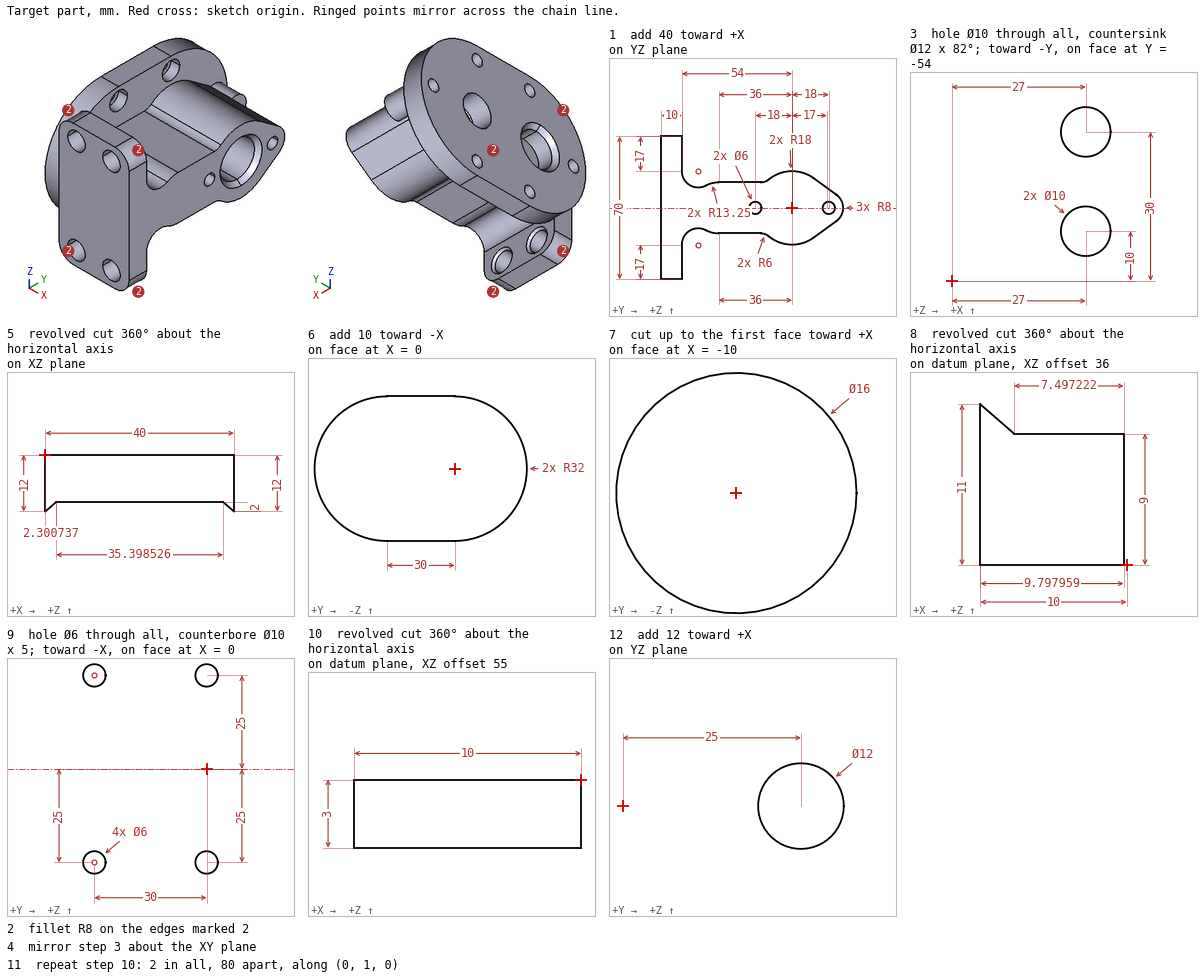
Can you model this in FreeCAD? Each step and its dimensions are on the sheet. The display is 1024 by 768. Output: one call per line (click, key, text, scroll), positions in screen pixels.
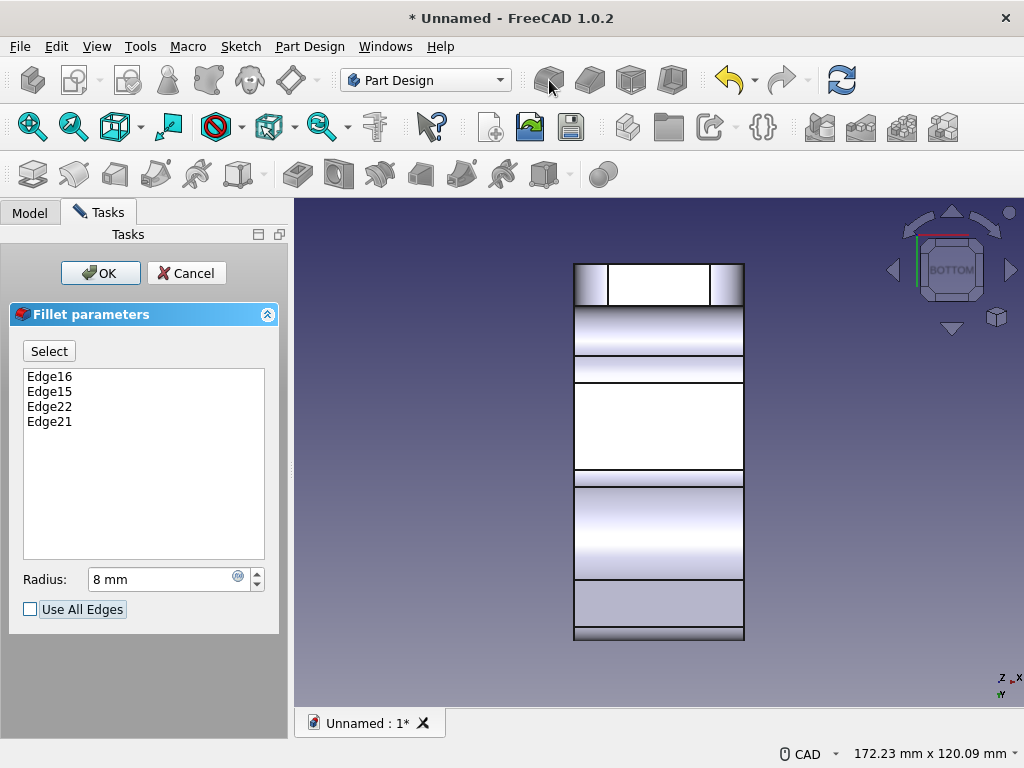
click(101, 273)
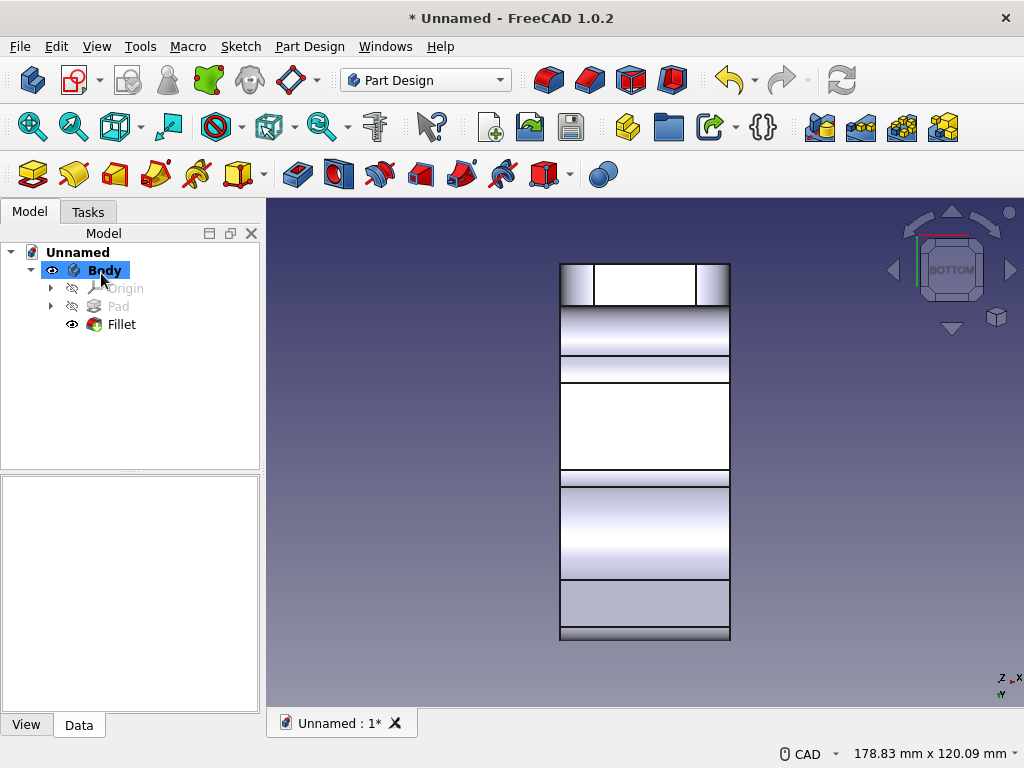
key(4)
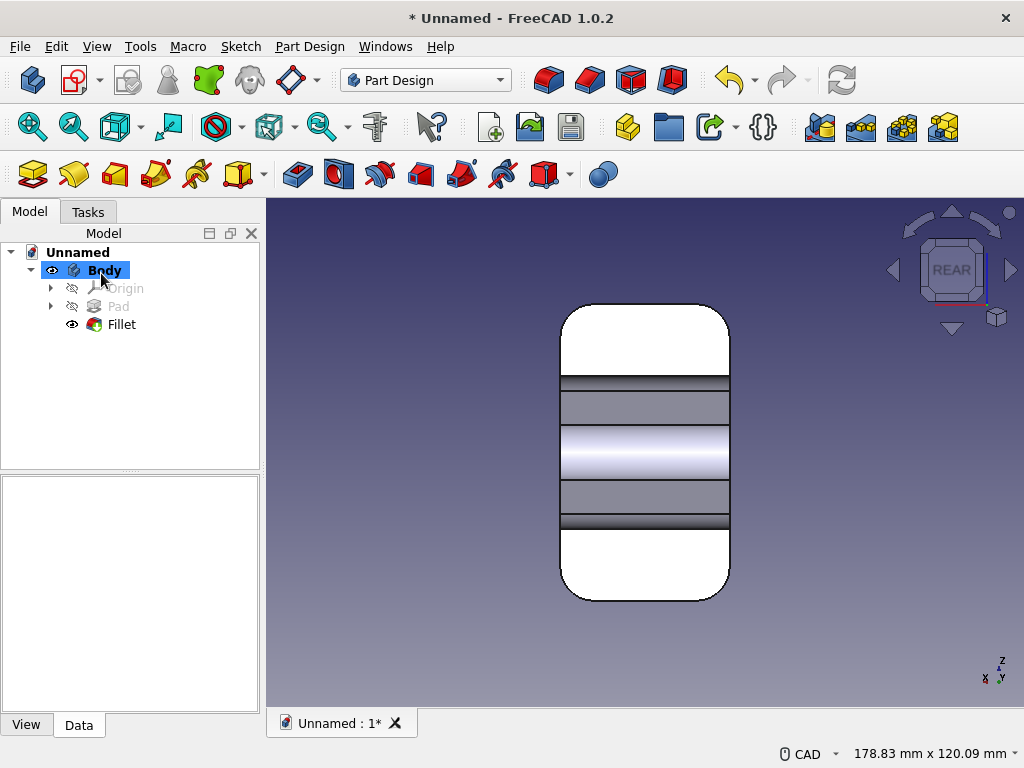
click(597, 564)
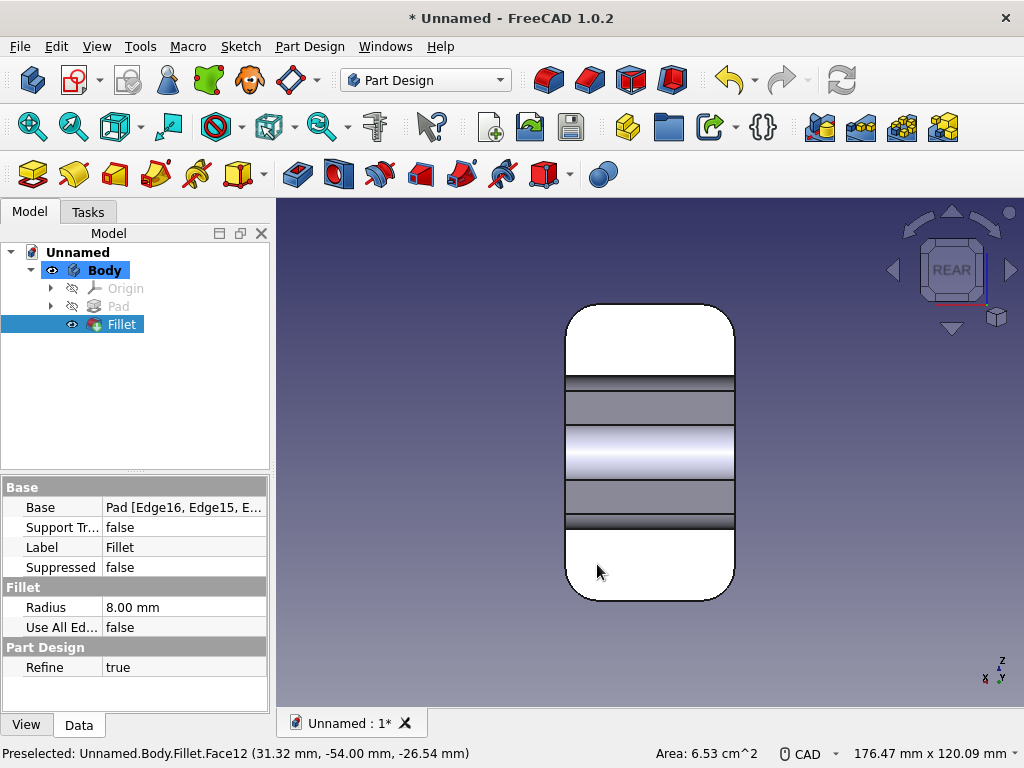
click(74, 80)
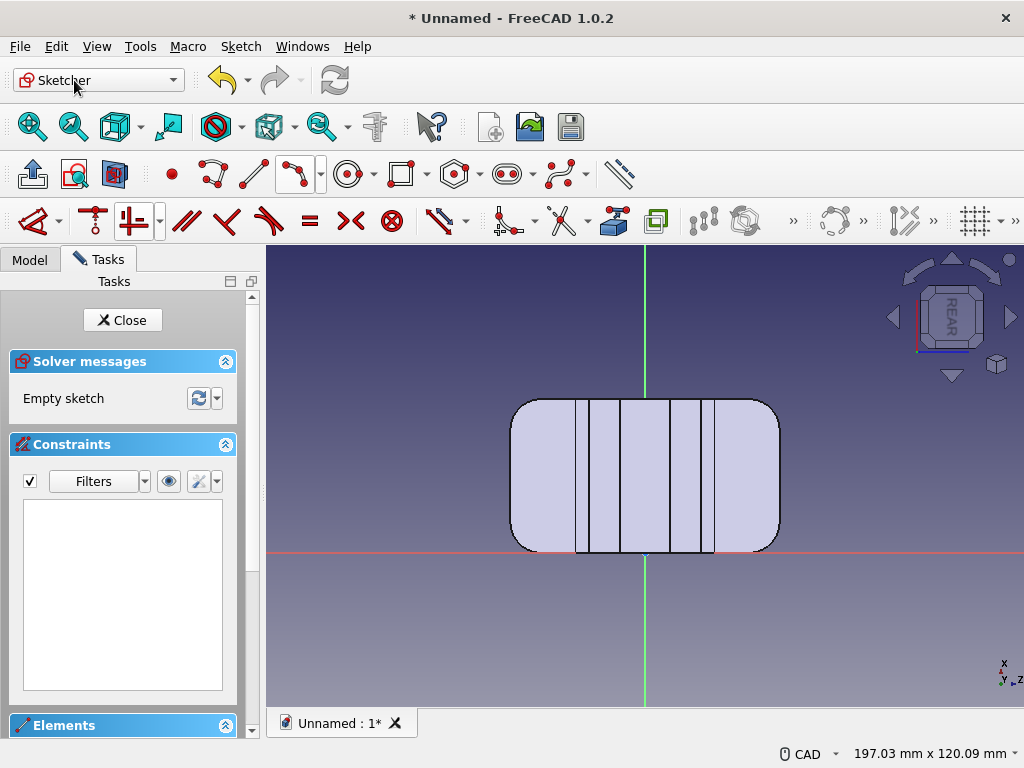
click(115, 174)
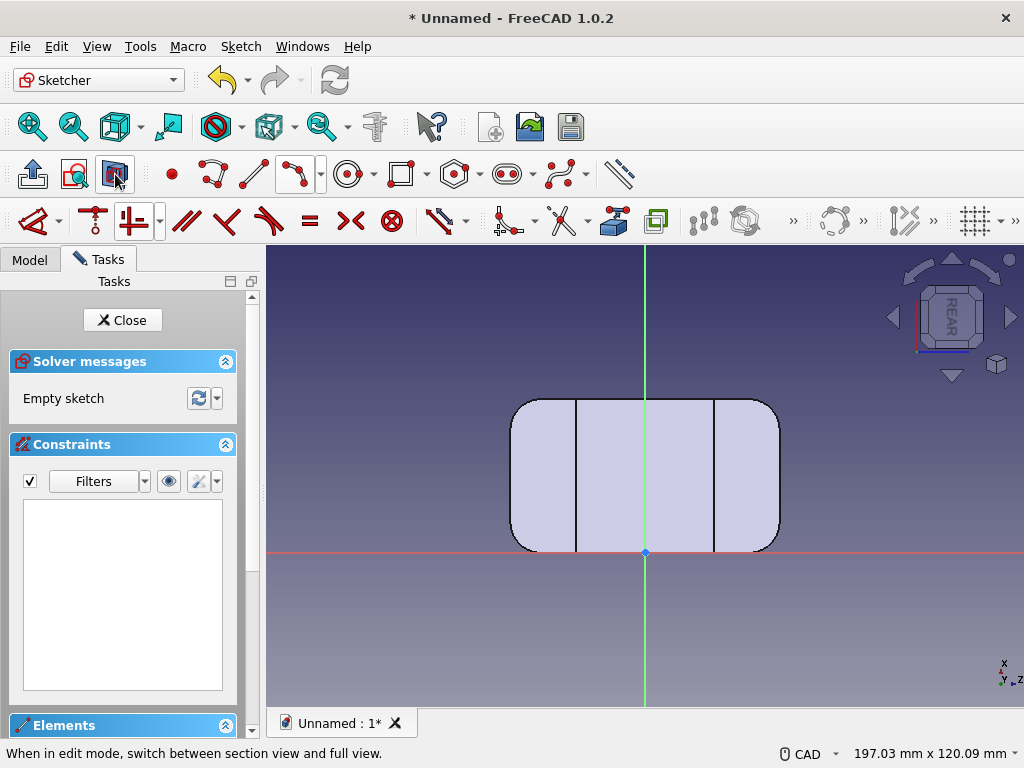
scroll(813, 493, up, 4)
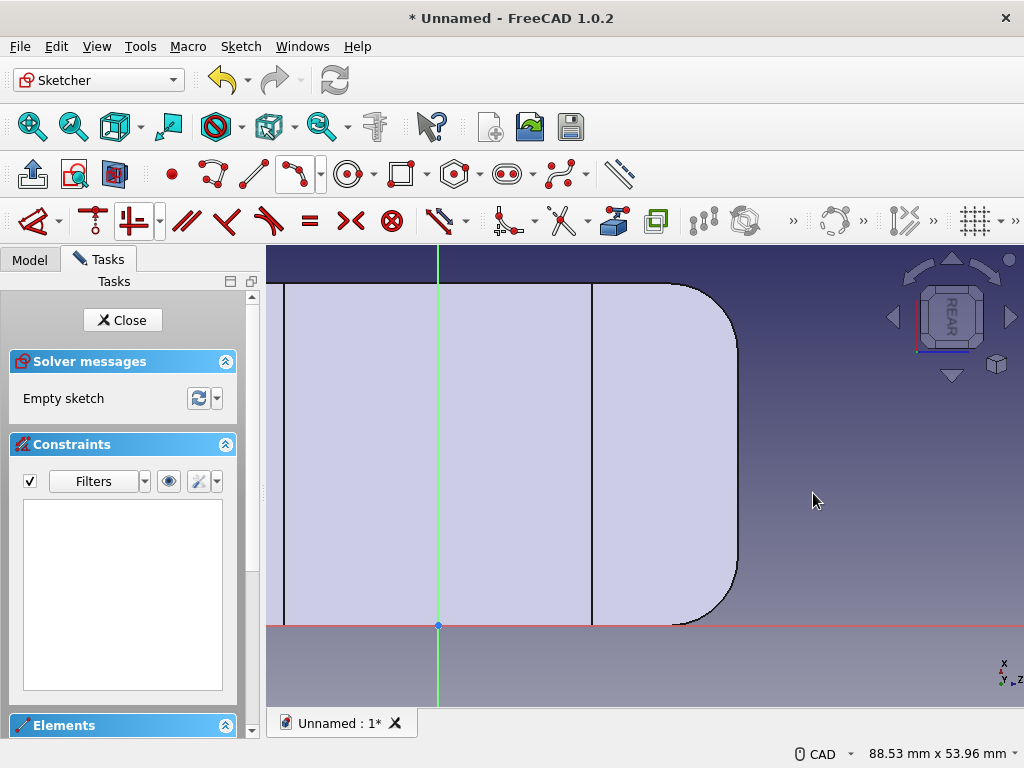
click(348, 174)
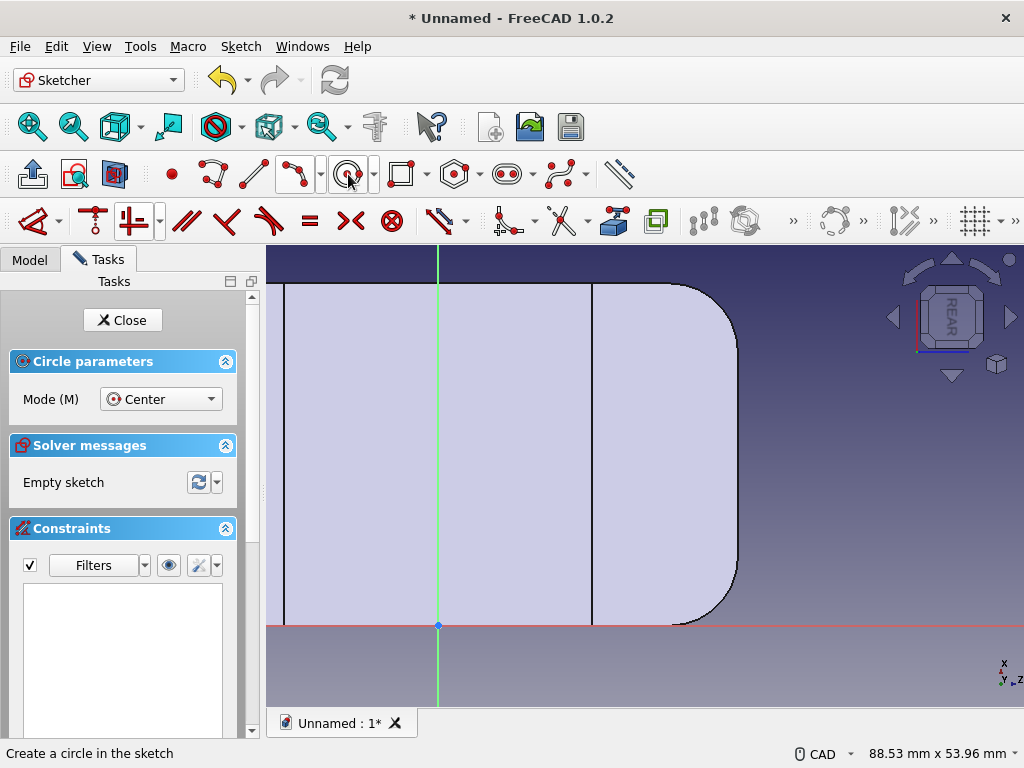
click(669, 540)
click(700, 510)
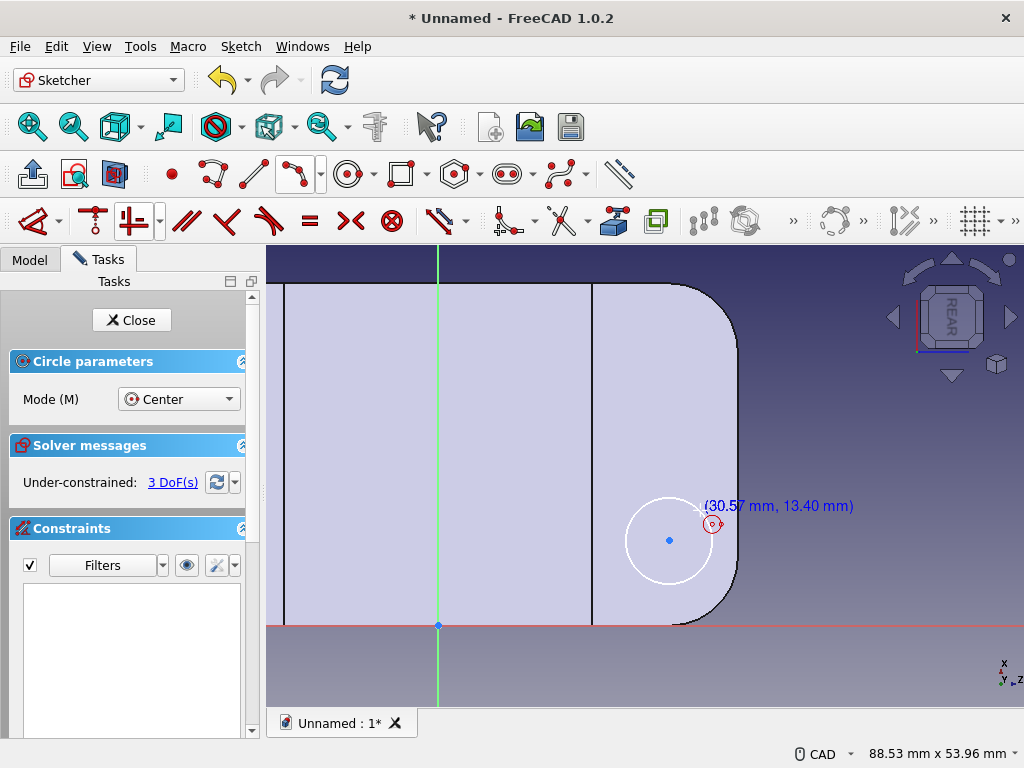
click(669, 369)
click(700, 339)
key(Escape)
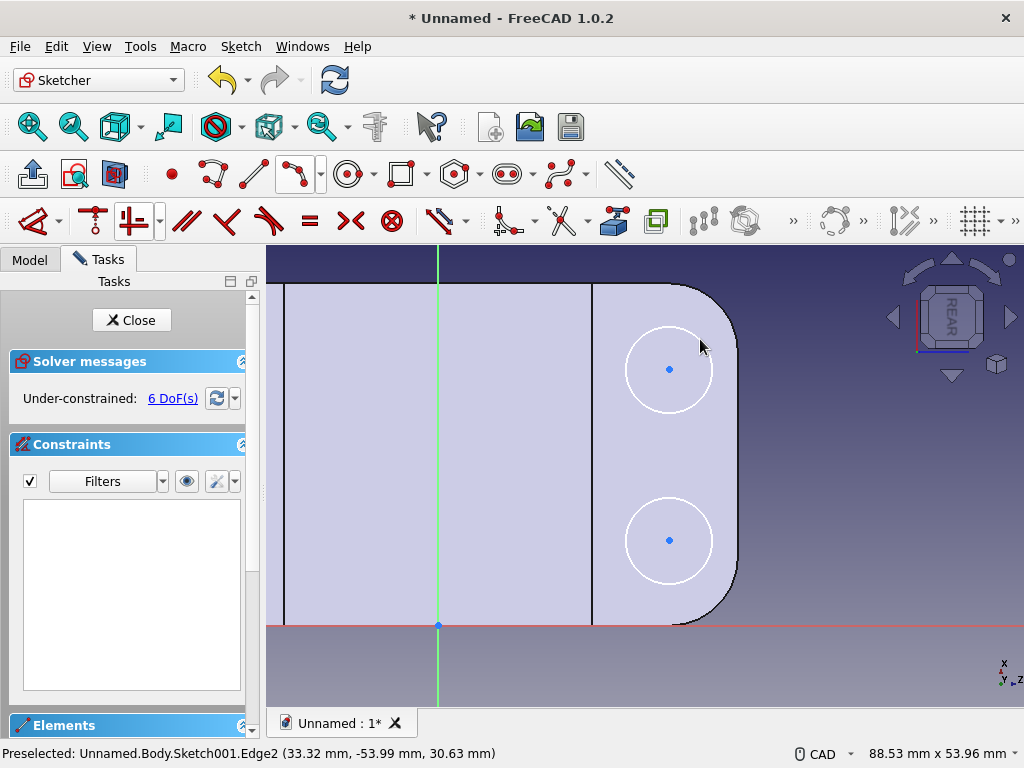
click(699, 510)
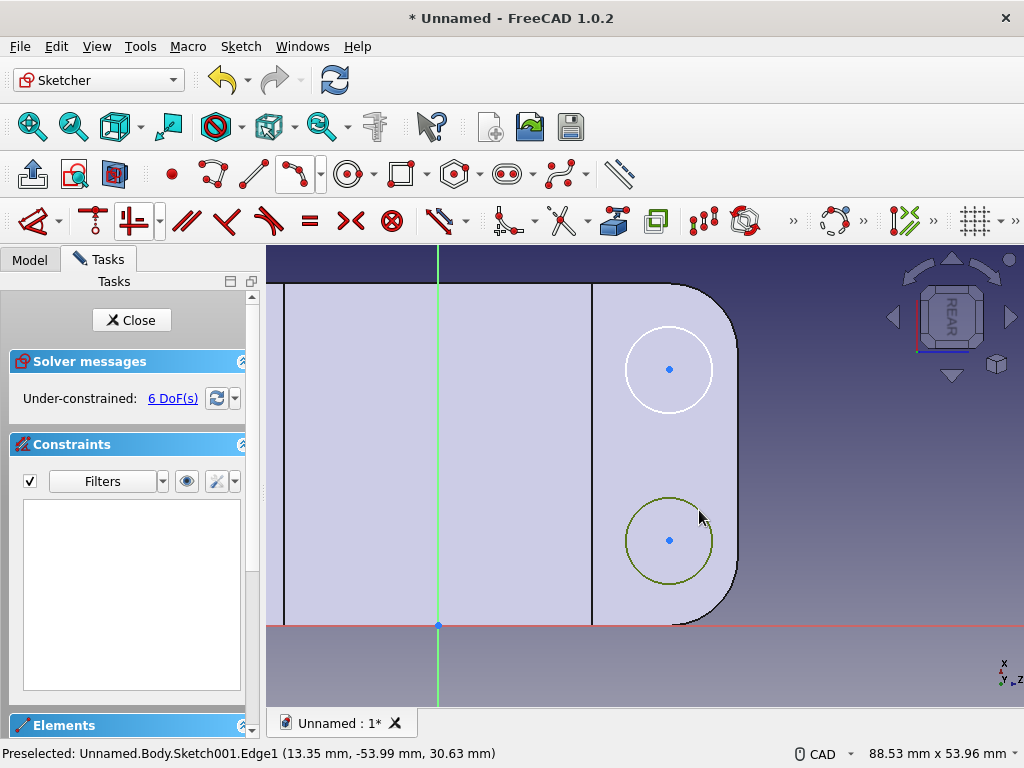
click(699, 339)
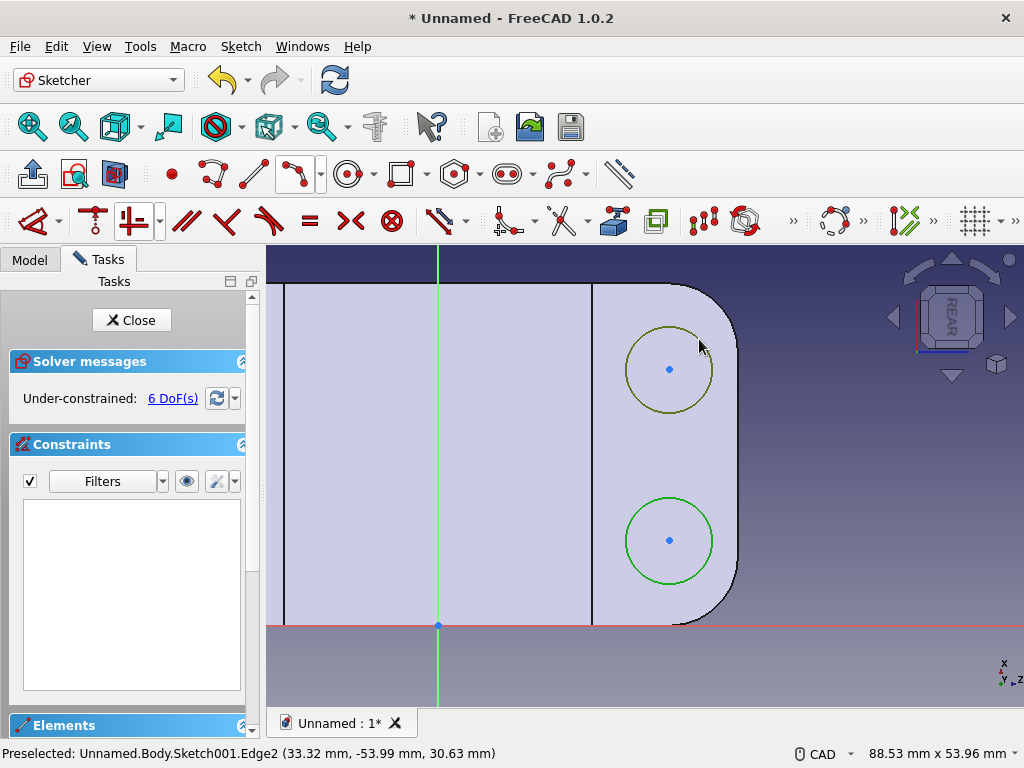
click(310, 222)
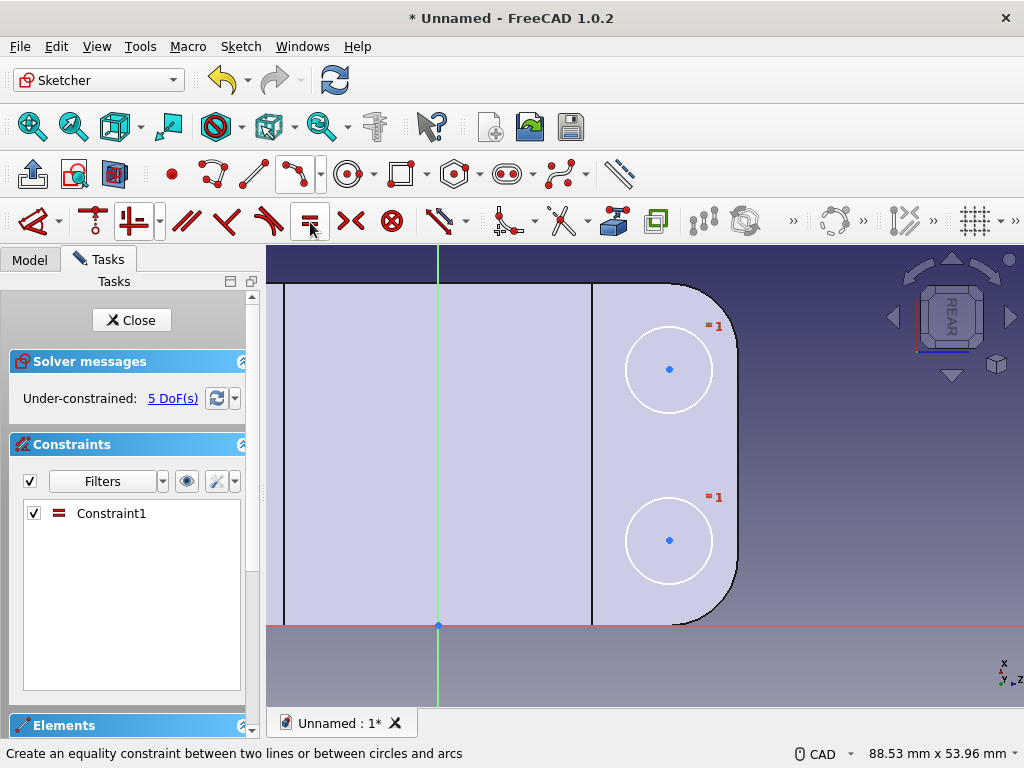
click(32, 222)